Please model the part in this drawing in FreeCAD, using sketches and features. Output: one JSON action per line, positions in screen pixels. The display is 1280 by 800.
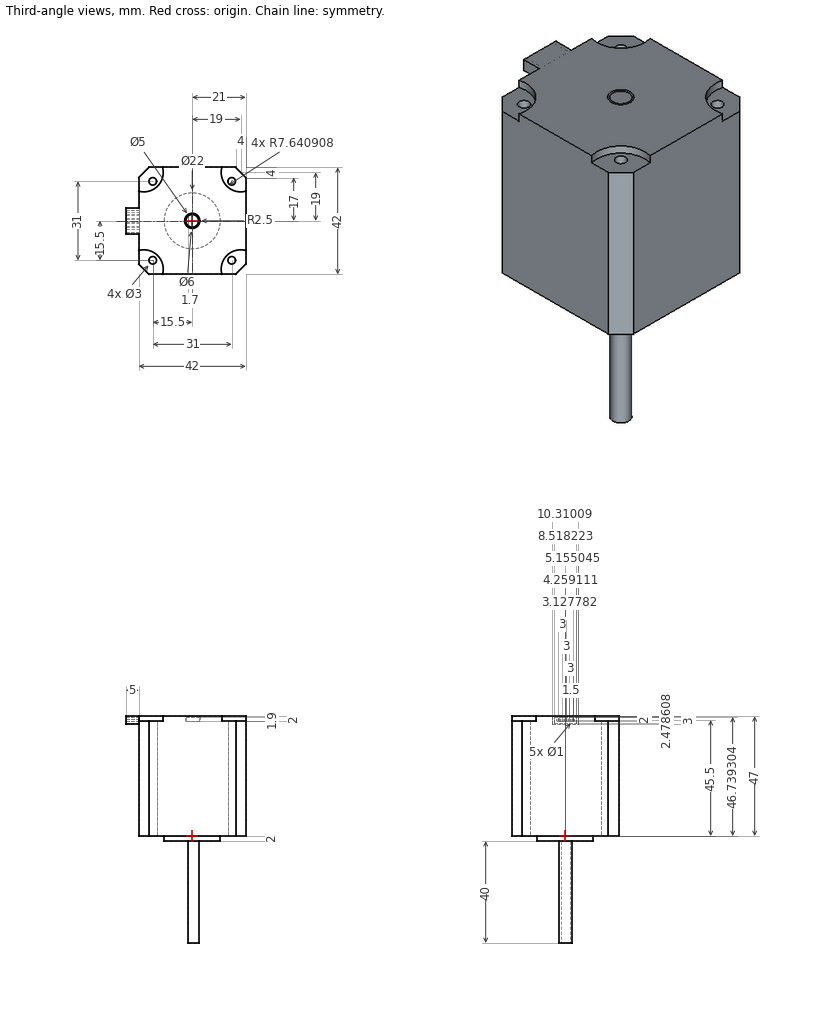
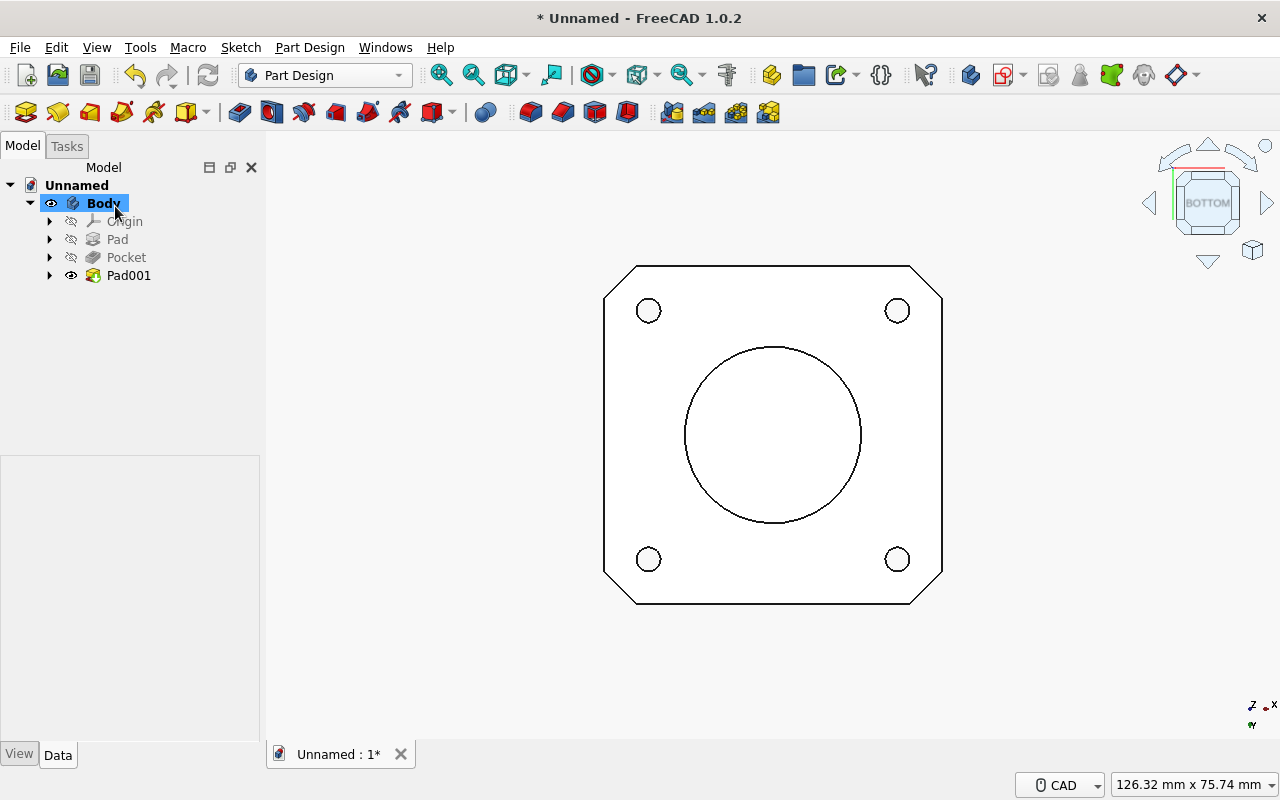
{"action": "left_click", "coordinate": [773, 434]}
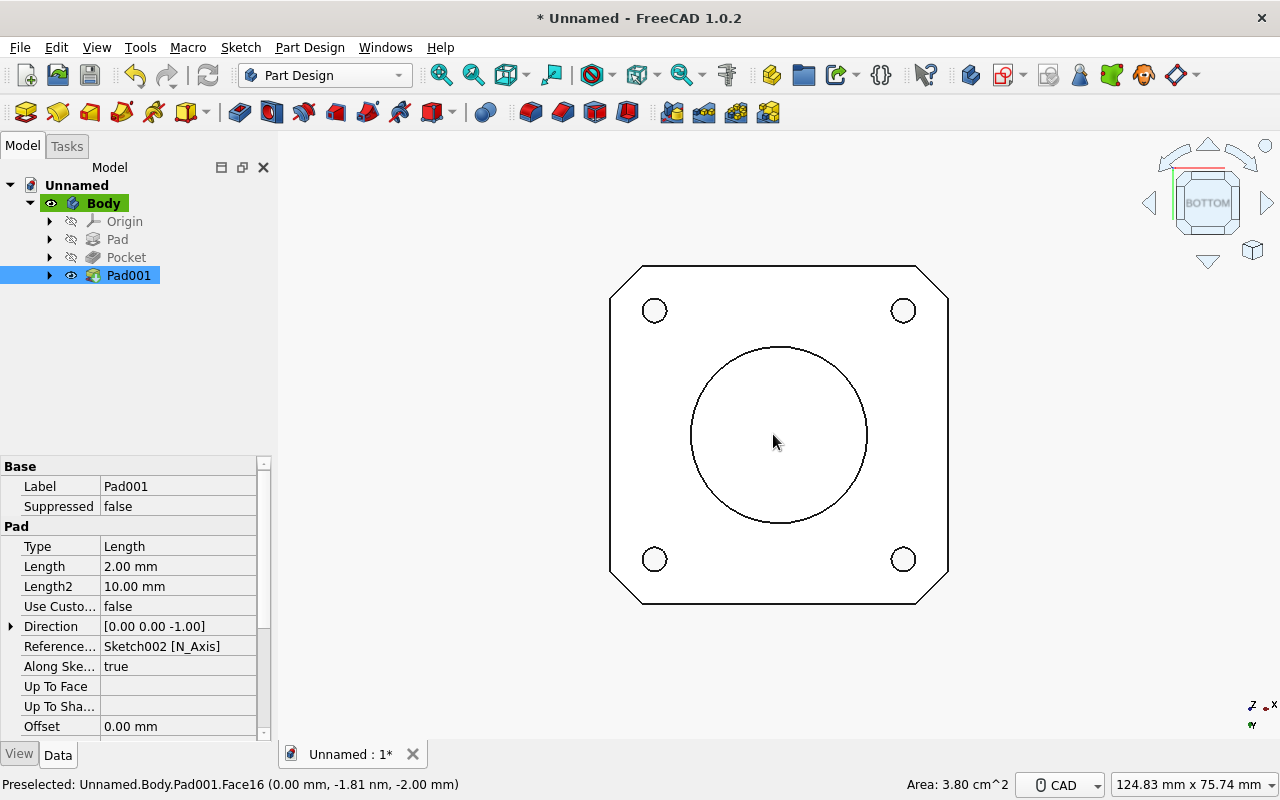
{"action": "left_click", "coordinate": [1004, 76]}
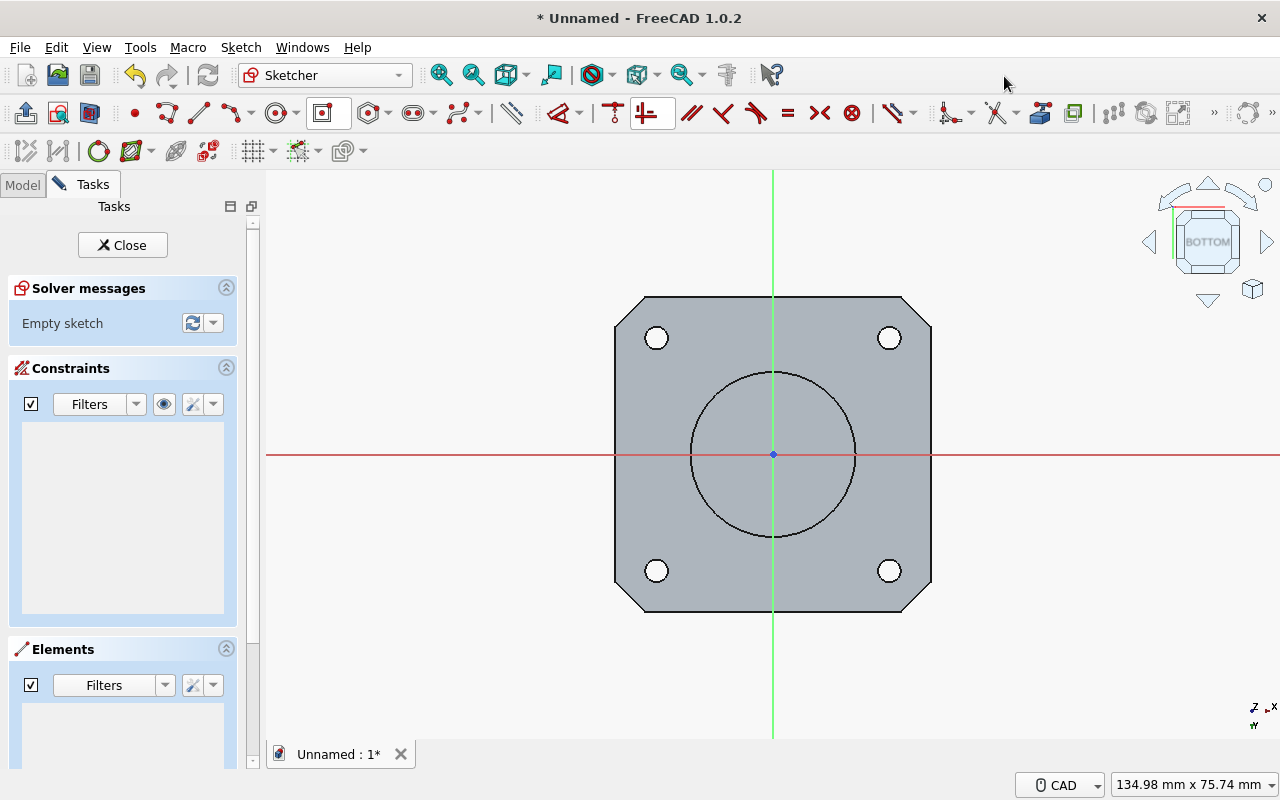
{"action": "scroll", "coordinate": [782, 455], "scroll_direction": "up", "scroll_amount": 13}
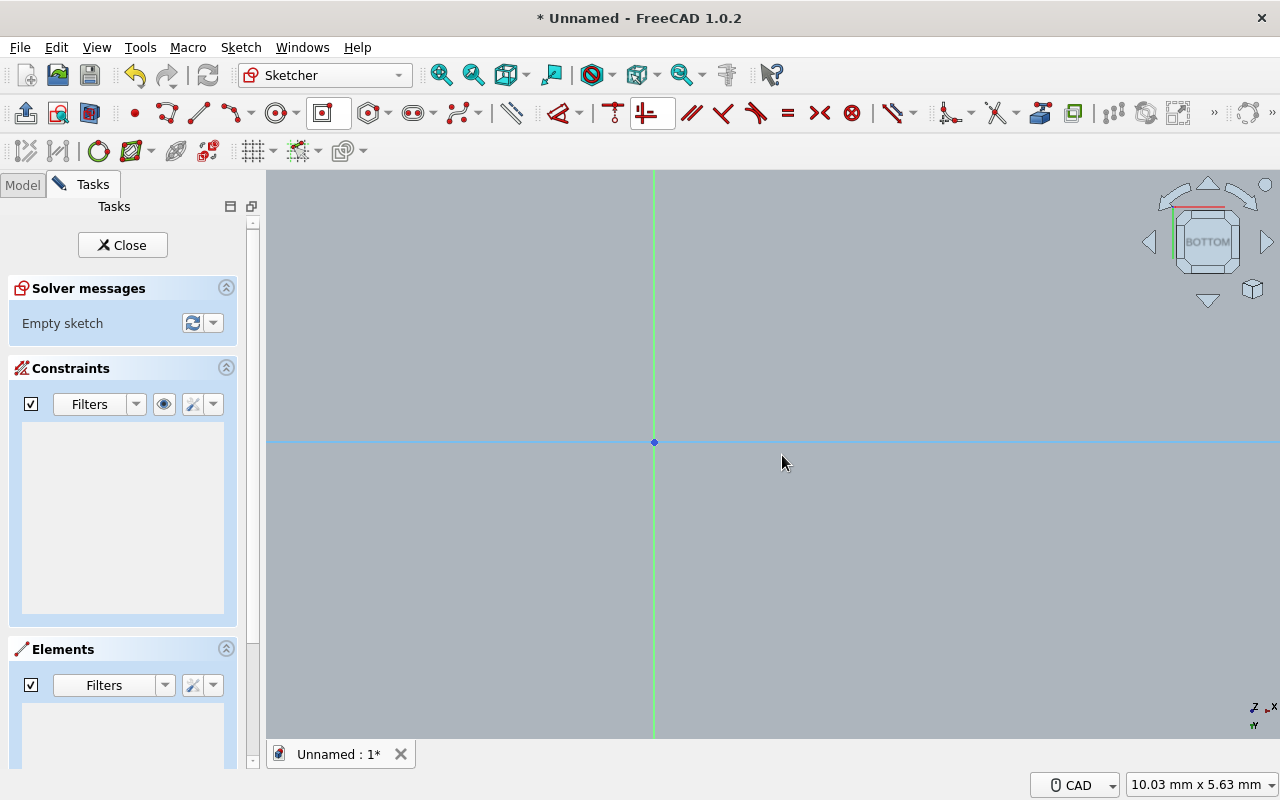
{"action": "key", "text": "g l"}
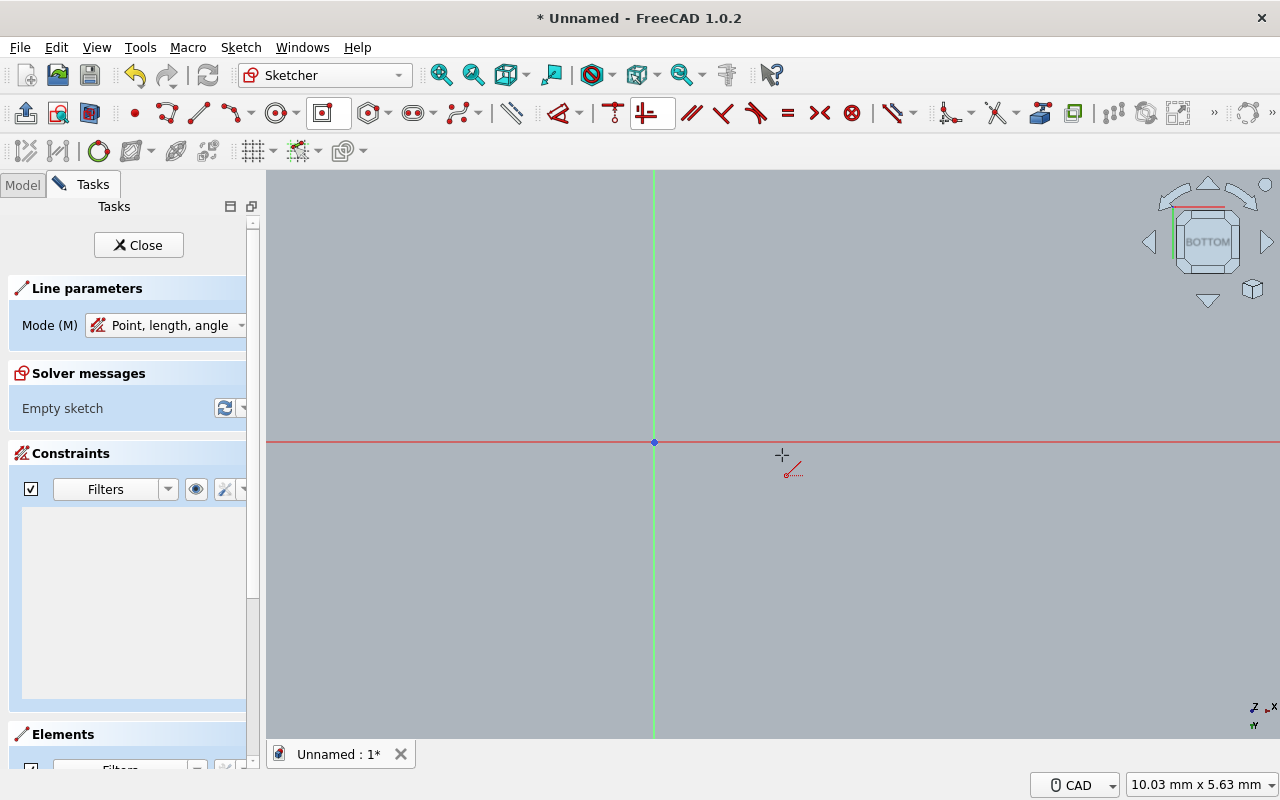
{"action": "left_click", "coordinate": [483, 257]}
{"action": "left_click", "coordinate": [483, 627]}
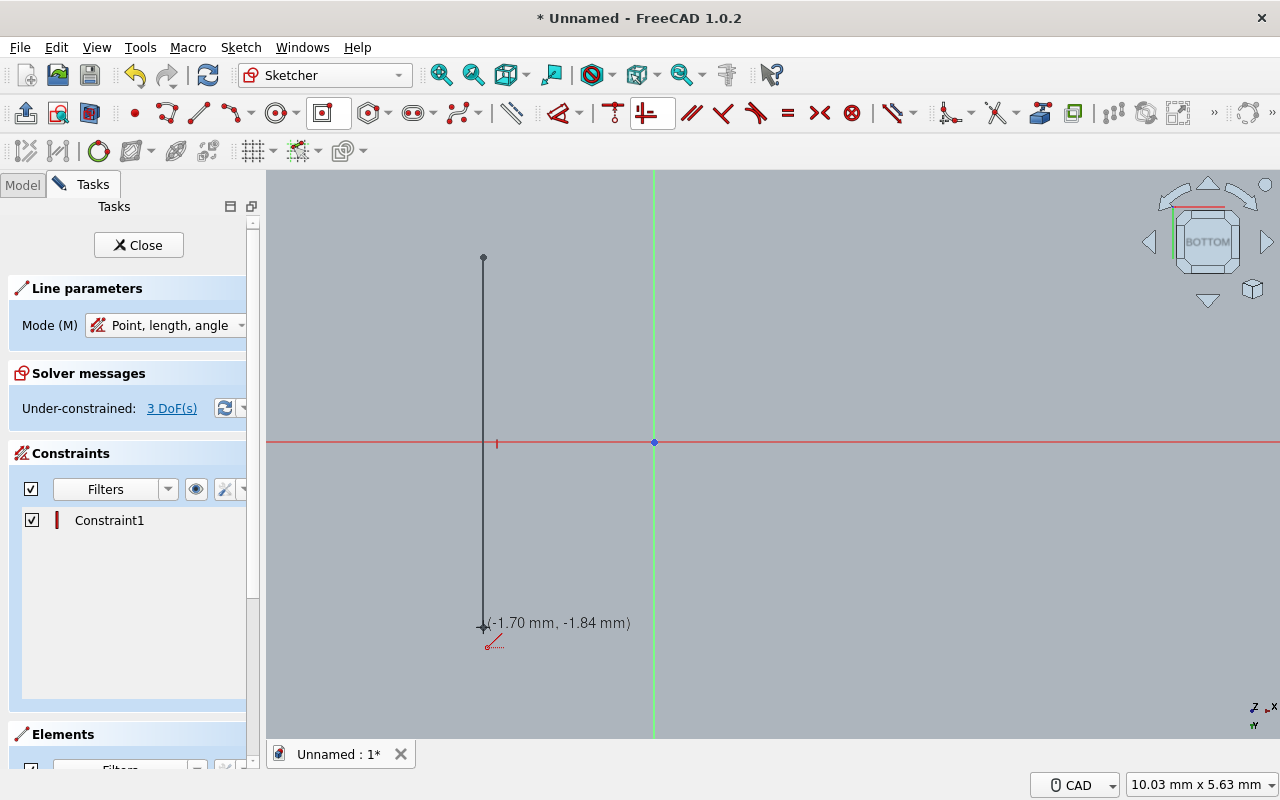
{"action": "left_click", "coordinate": [232, 114]}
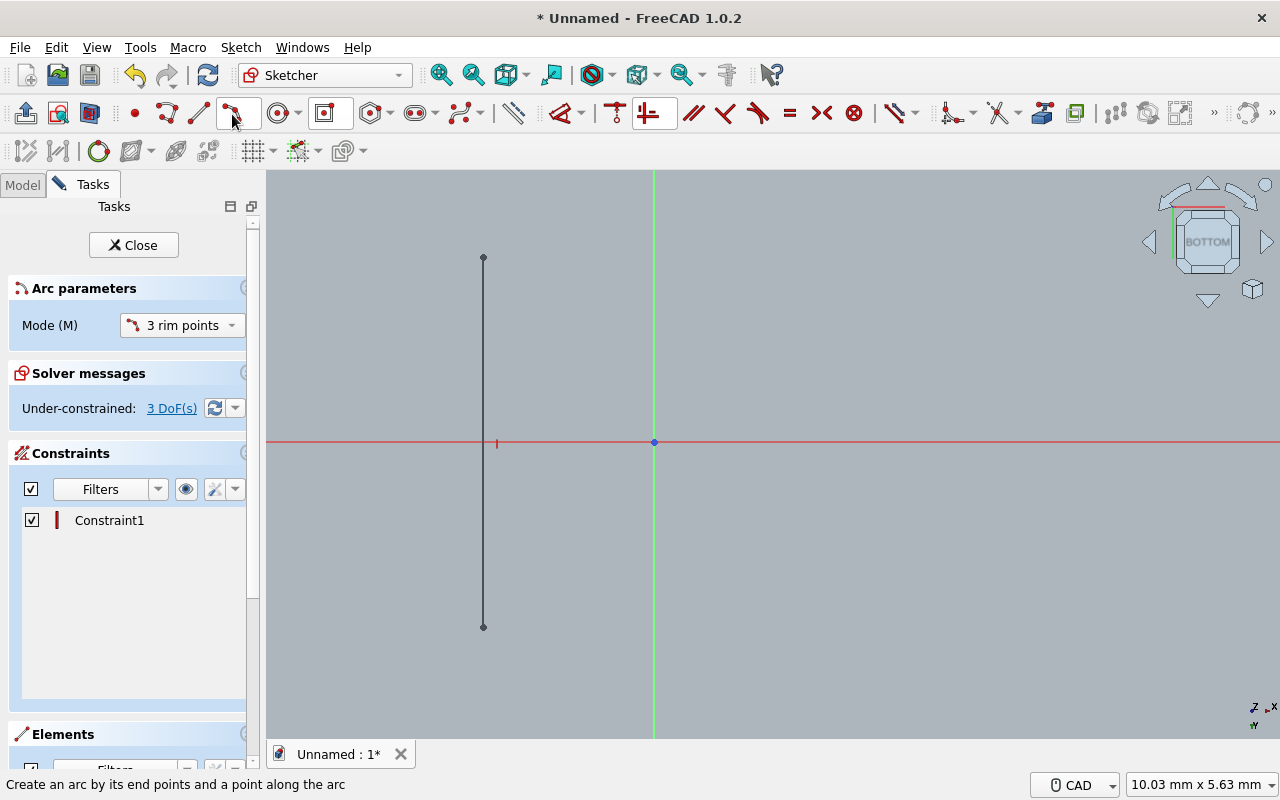
{"action": "left_click", "coordinate": [483, 628]}
{"action": "left_click", "coordinate": [483, 258]}
{"action": "left_click", "coordinate": [881, 555]}
{"action": "key", "text": "Escape"}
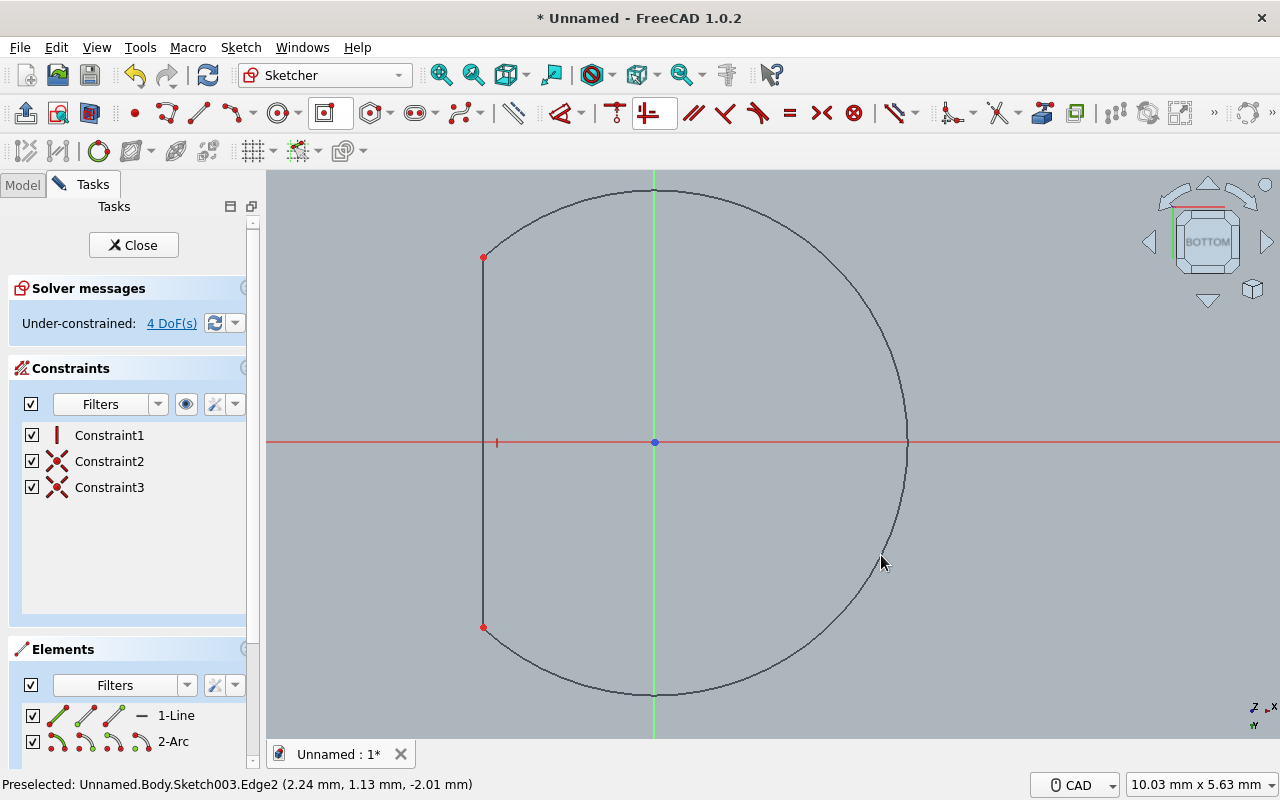
{"action": "left_click_drag", "start_coordinate": [644, 432], "coordinate": [665, 453]}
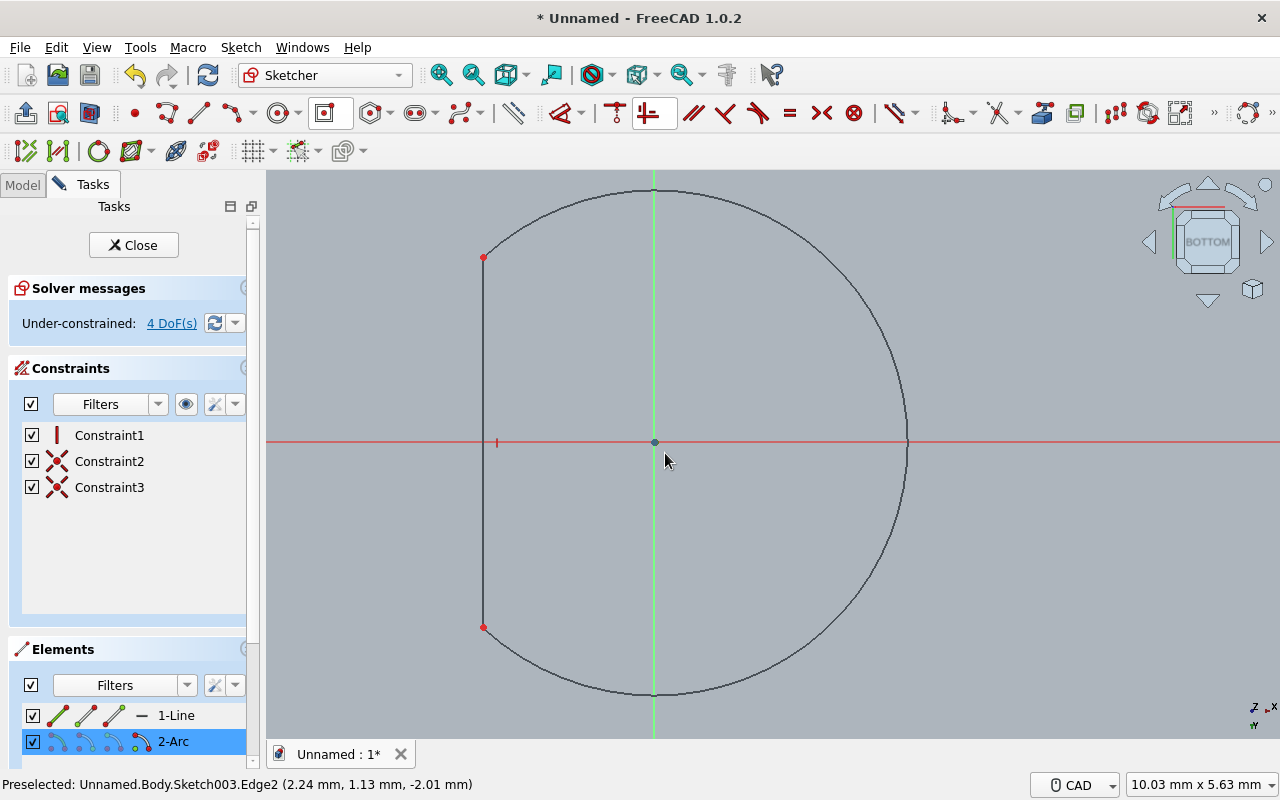
{"action": "left_click", "coordinate": [616, 114]}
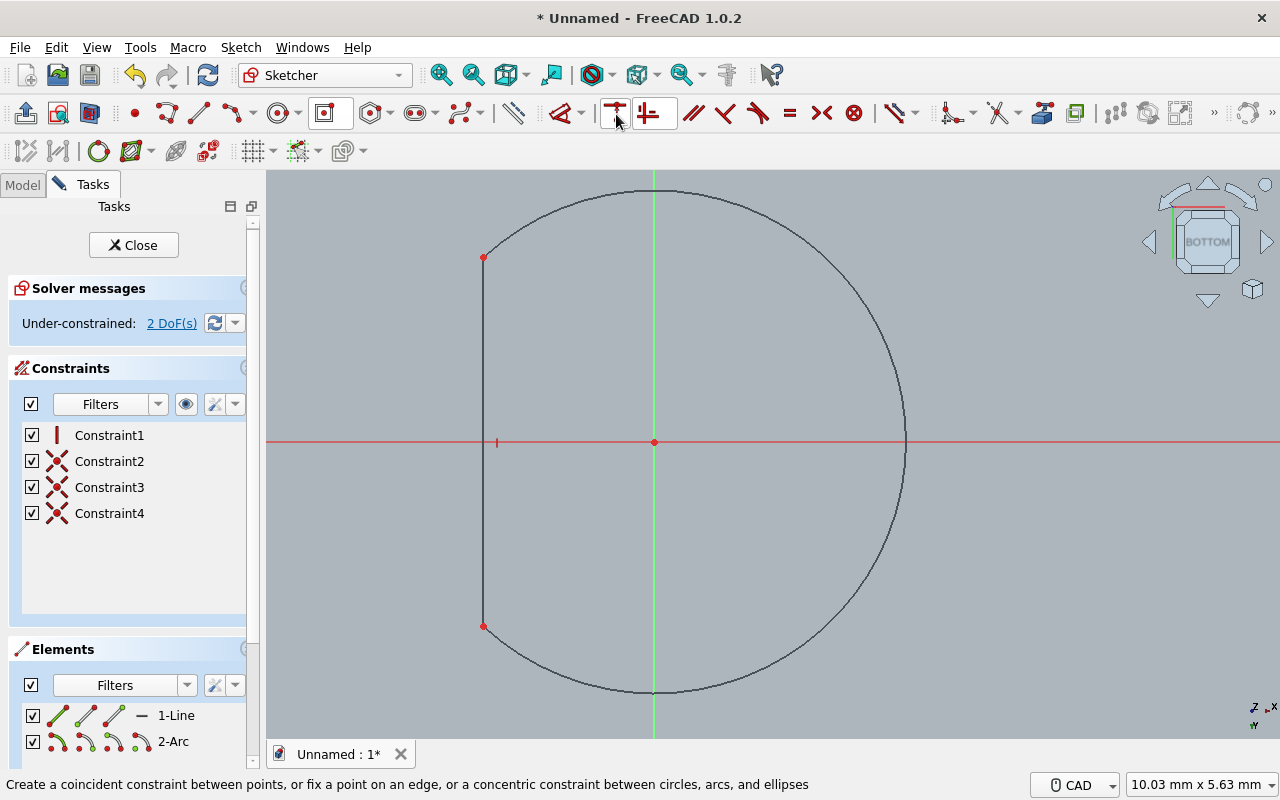
{"action": "left_click", "coordinate": [560, 114]}